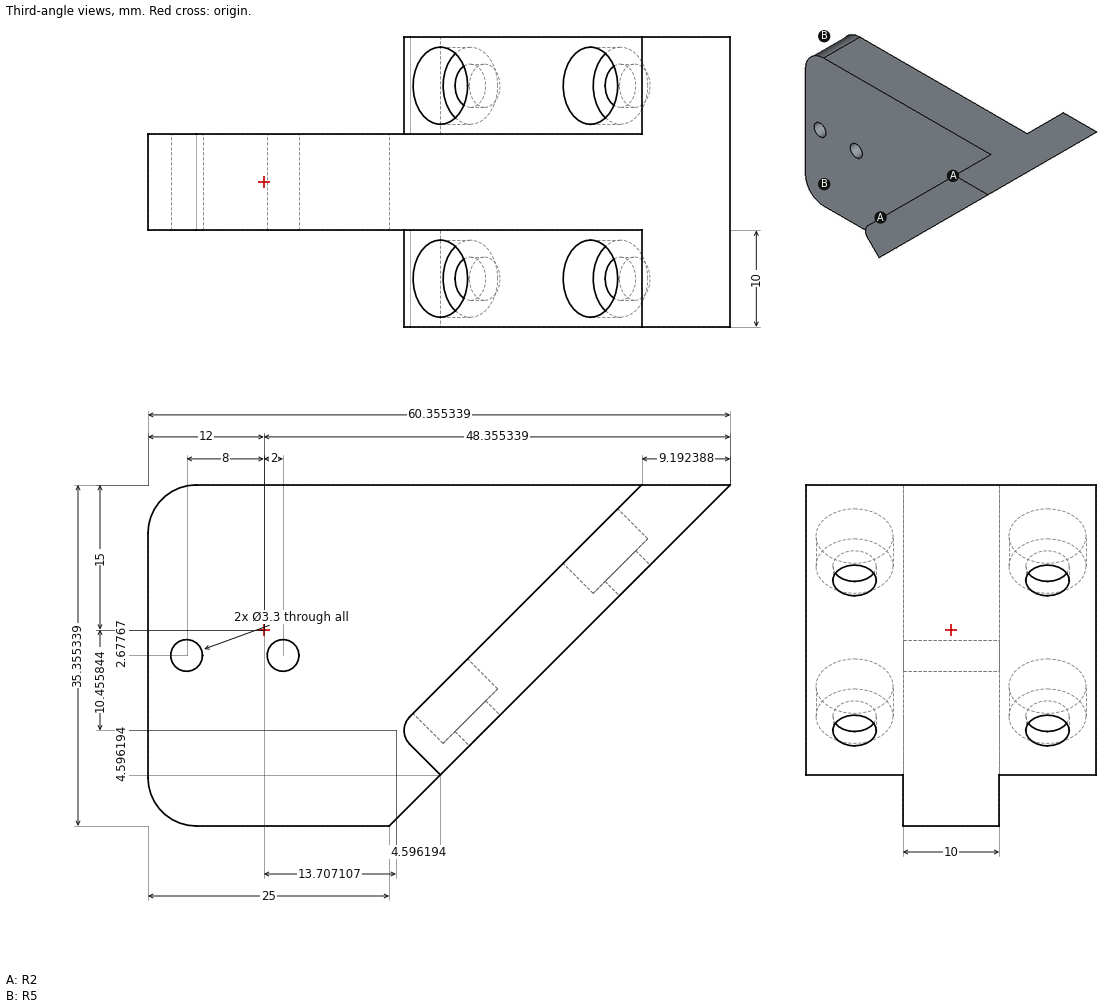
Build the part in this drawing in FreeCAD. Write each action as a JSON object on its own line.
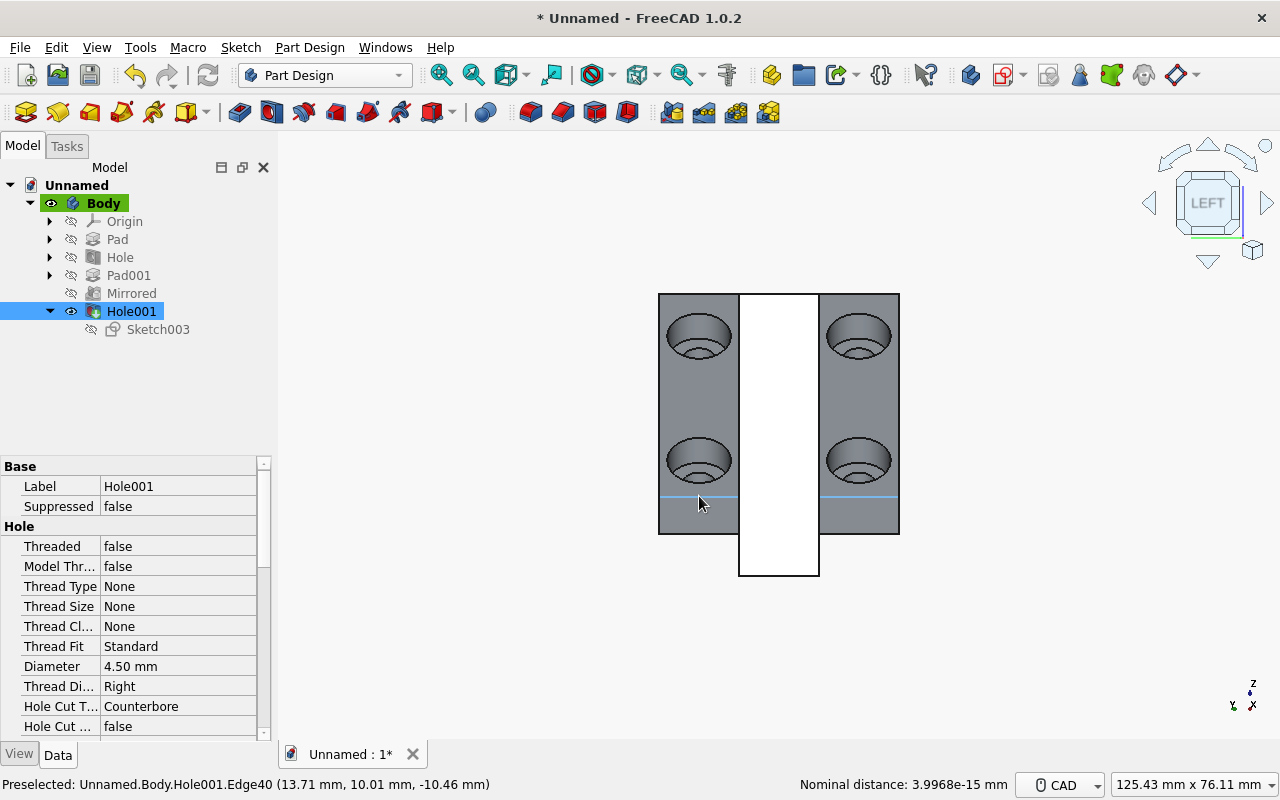
{"action": "left_click", "coordinate": [532, 112]}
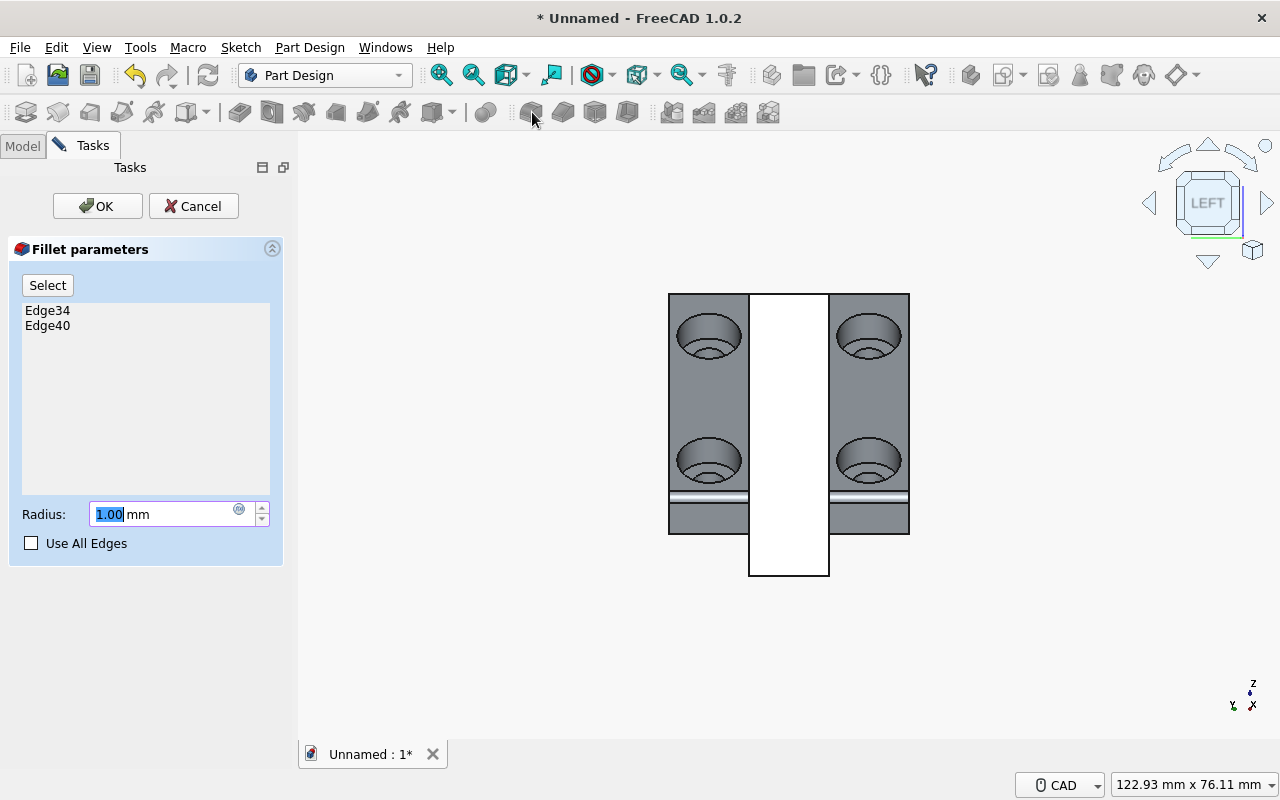
{"action": "type", "text": "2"}
{"action": "key", "text": "Tab"}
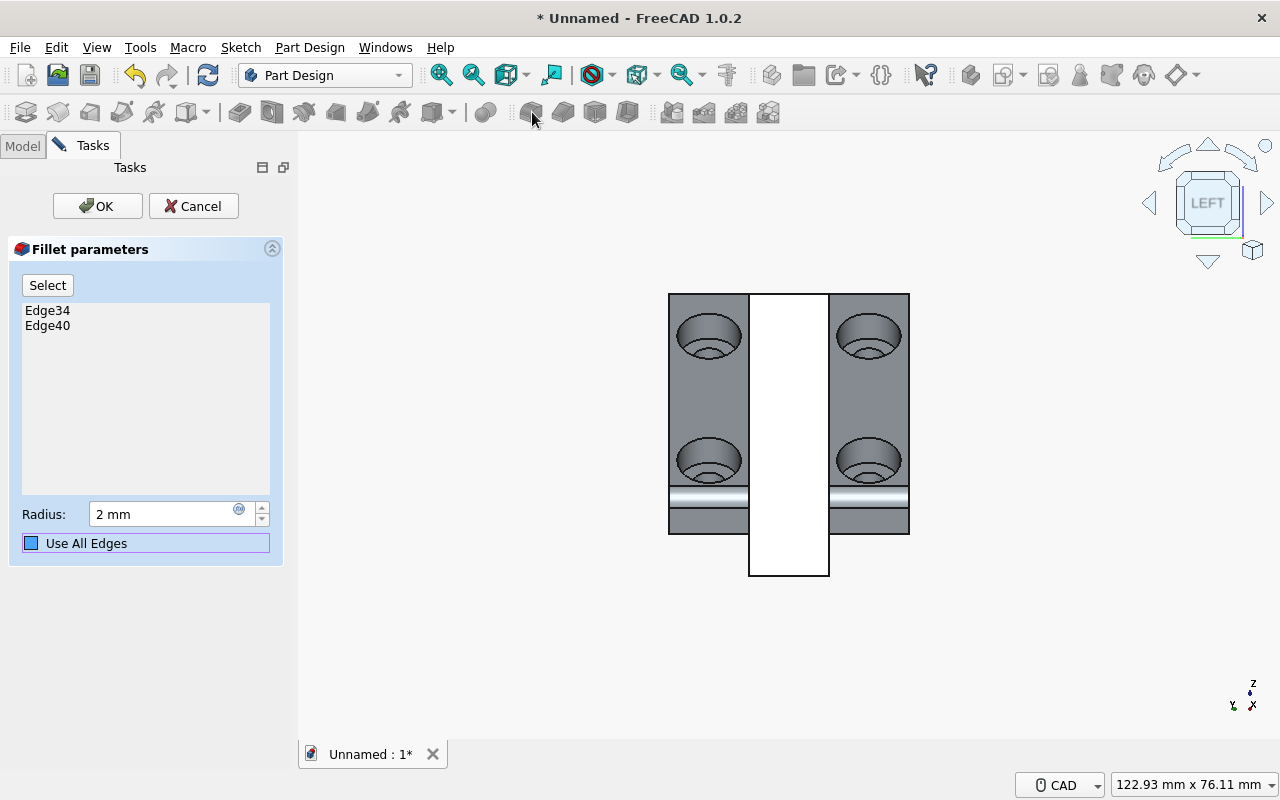
{"action": "left_click", "coordinate": [98, 206]}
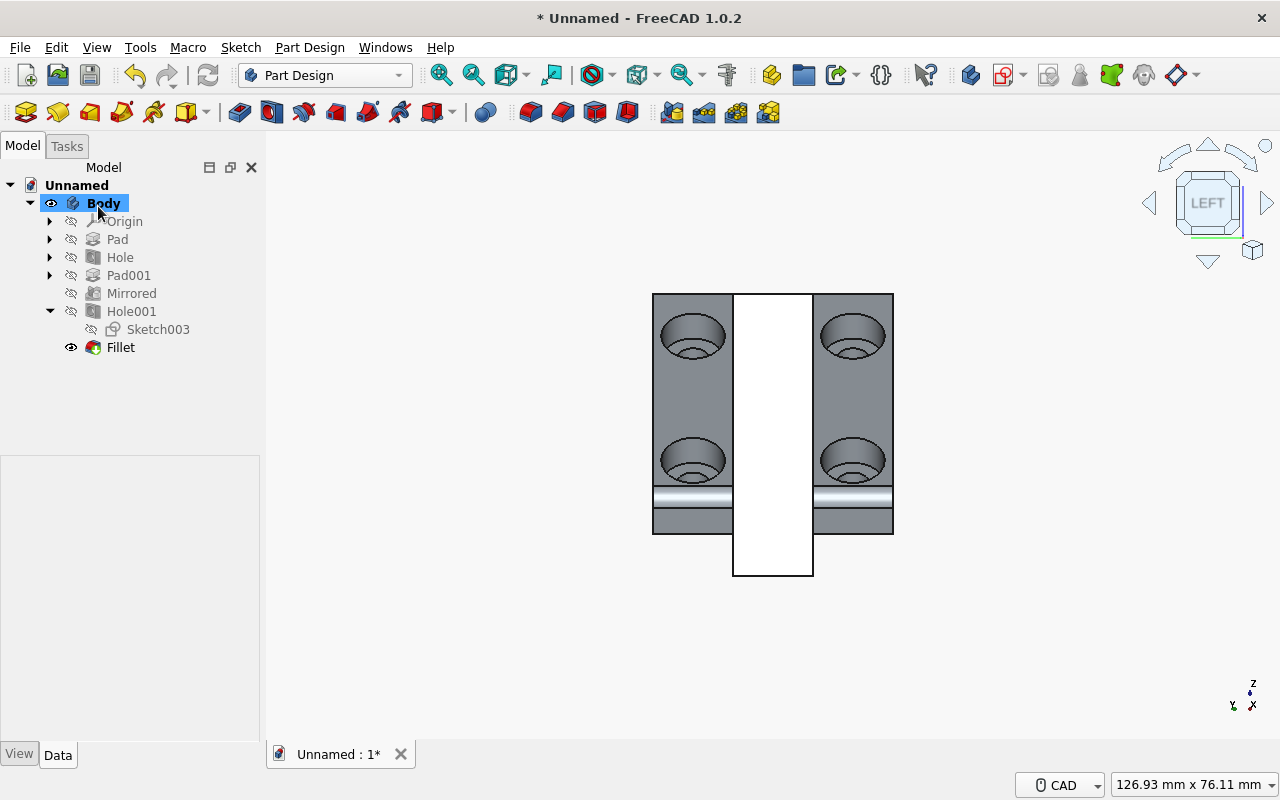
{"action": "left_click", "coordinate": [773, 293]}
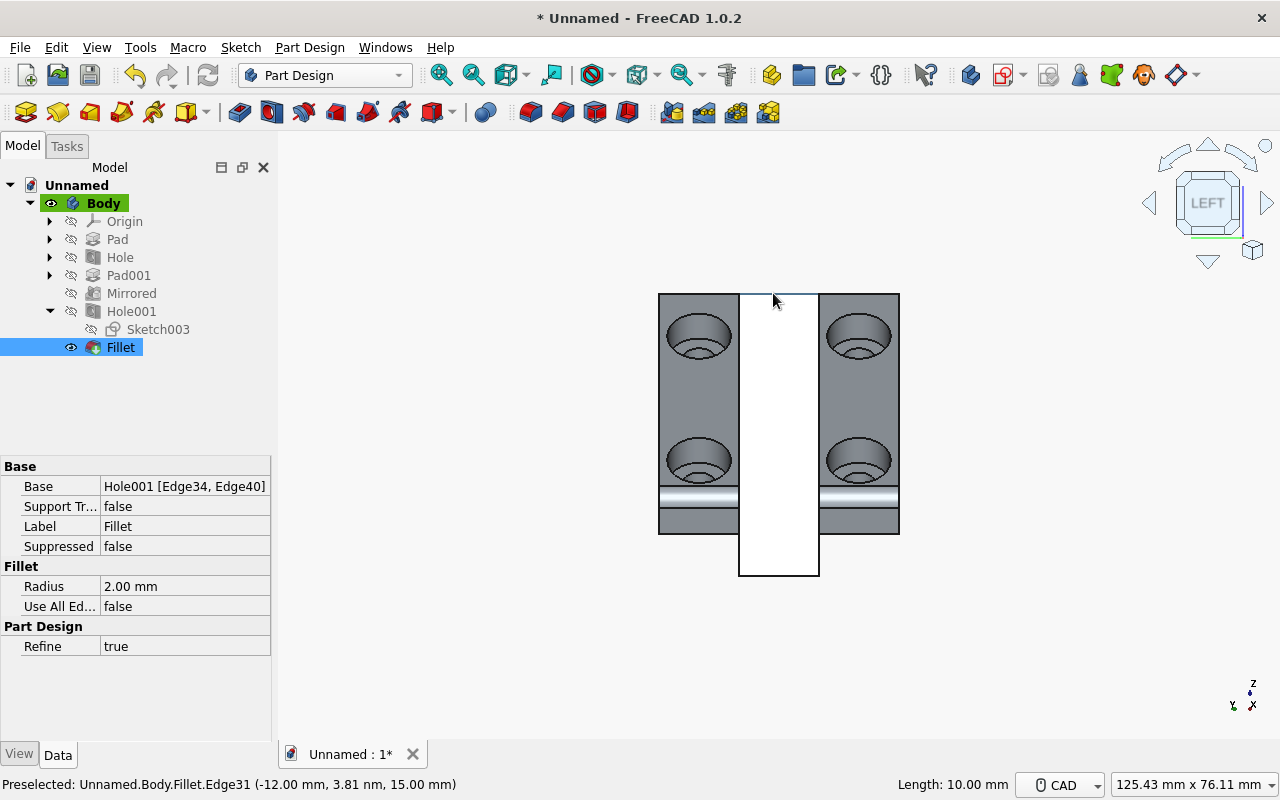
{"action": "left_click", "coordinate": [779, 575], "text": "ctrl"}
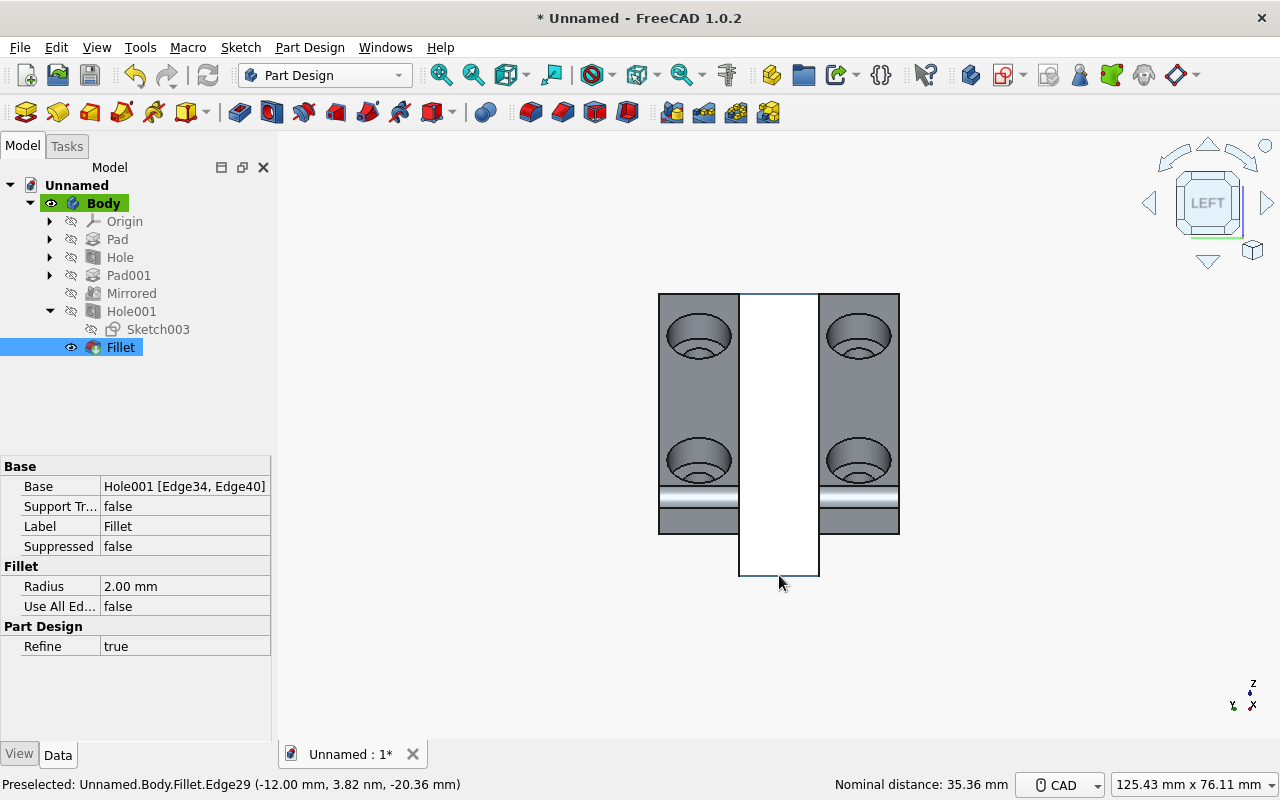
{"action": "left_click", "coordinate": [532, 112]}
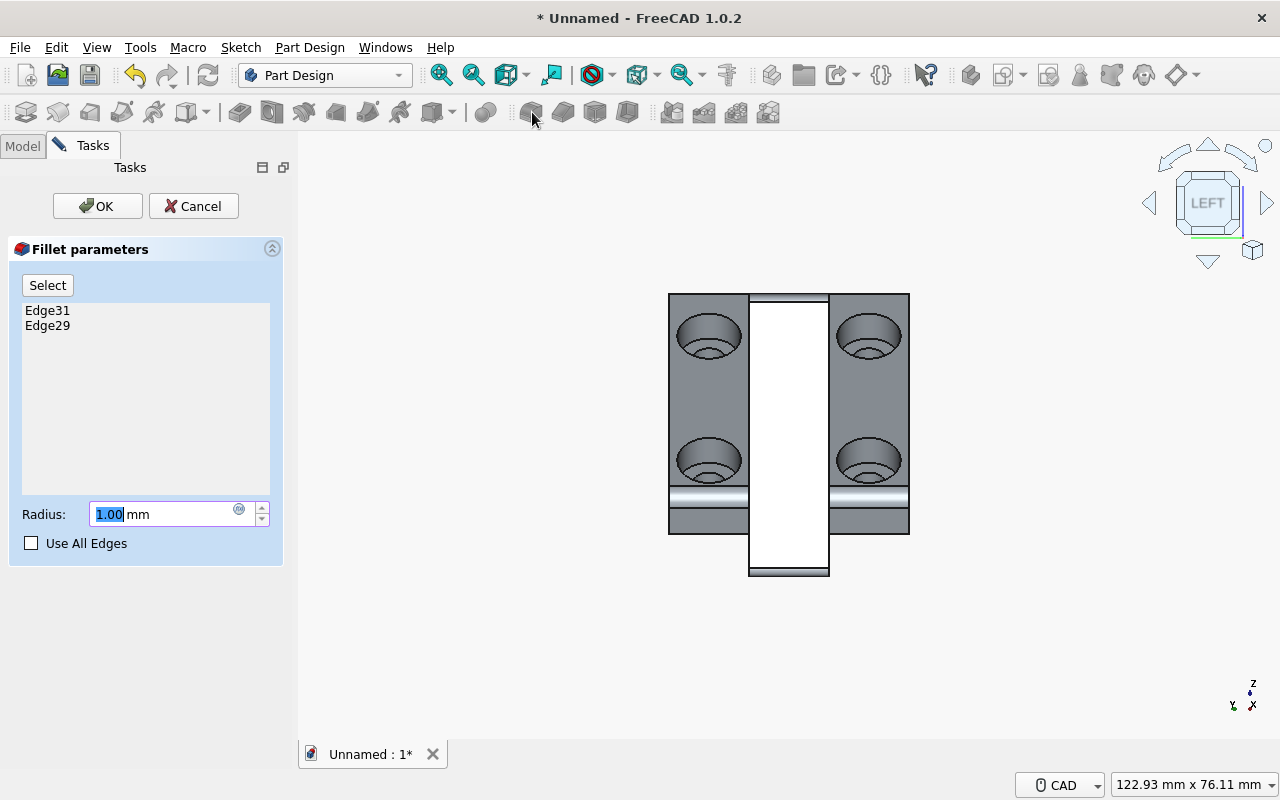
{"action": "type", "text": "5"}
{"action": "key", "text": "Tab"}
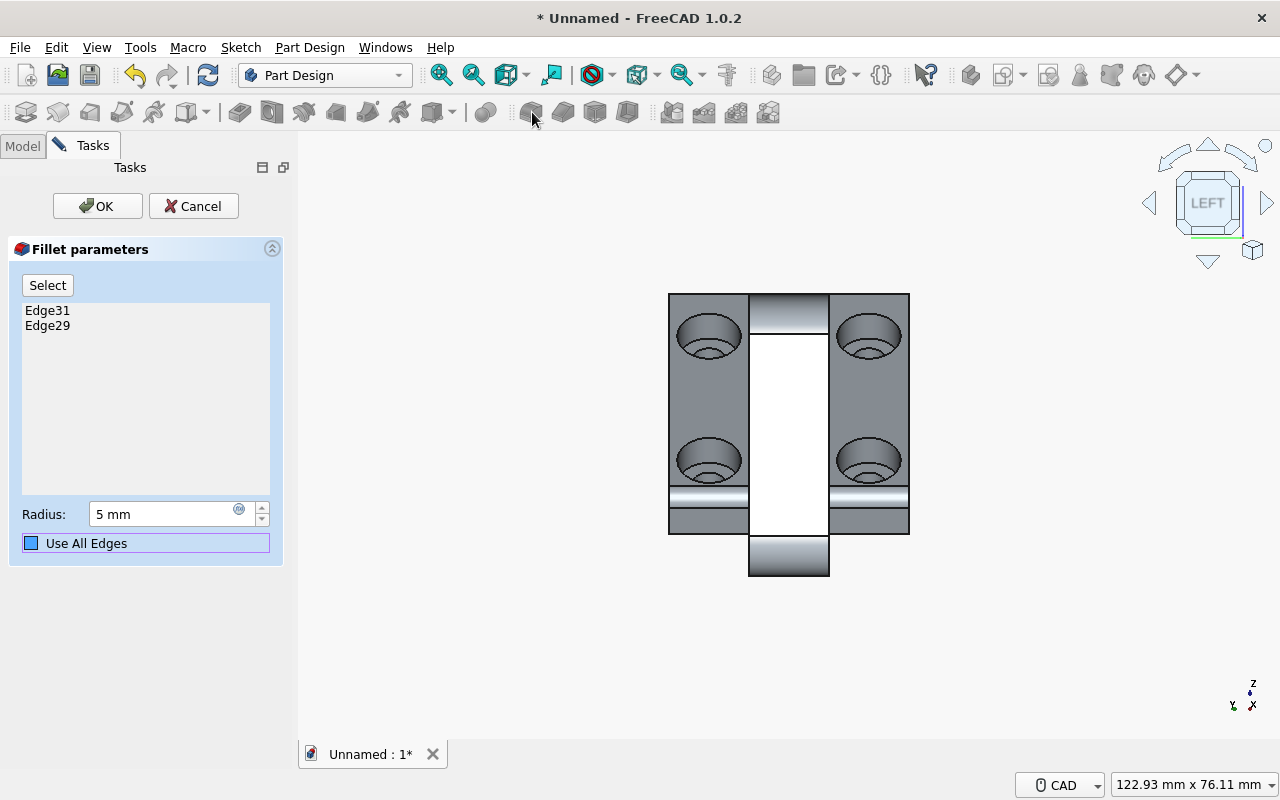
{"action": "left_click", "coordinate": [98, 206]}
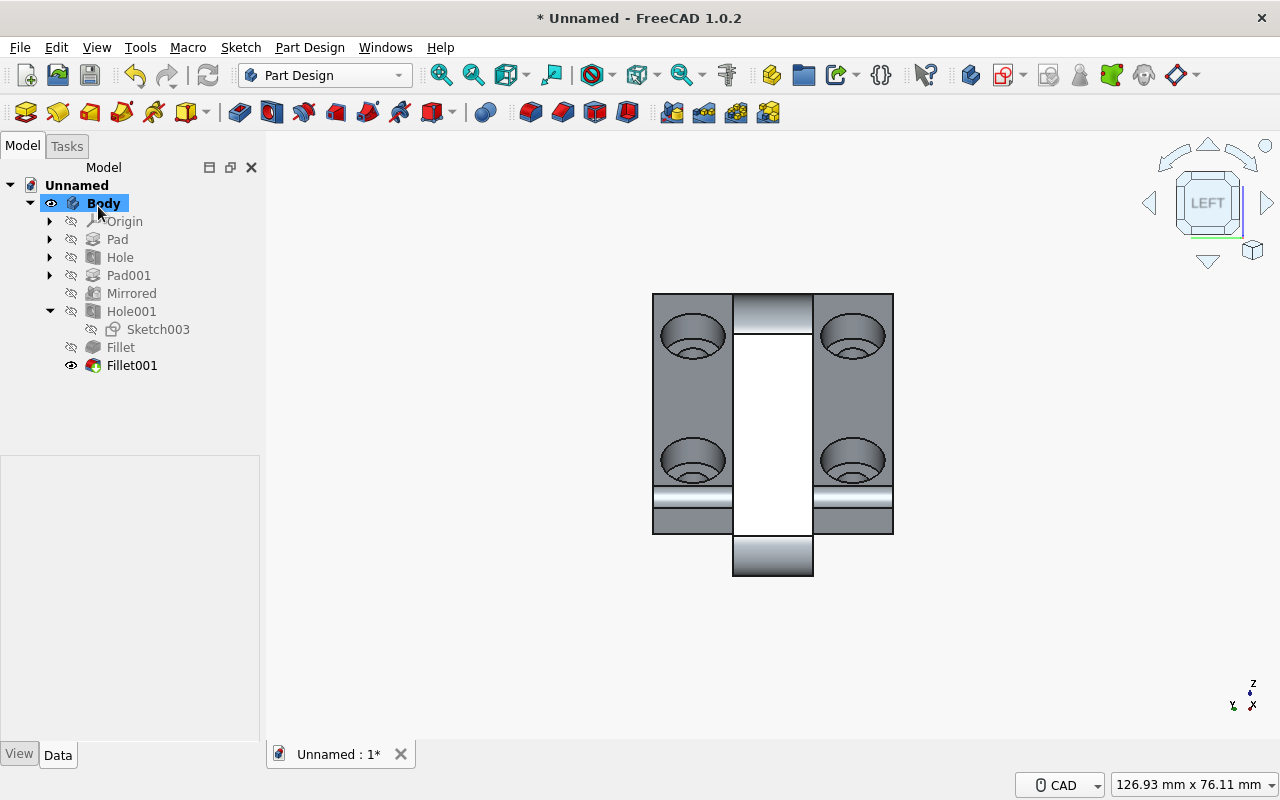
{"action": "key", "text": "0"}